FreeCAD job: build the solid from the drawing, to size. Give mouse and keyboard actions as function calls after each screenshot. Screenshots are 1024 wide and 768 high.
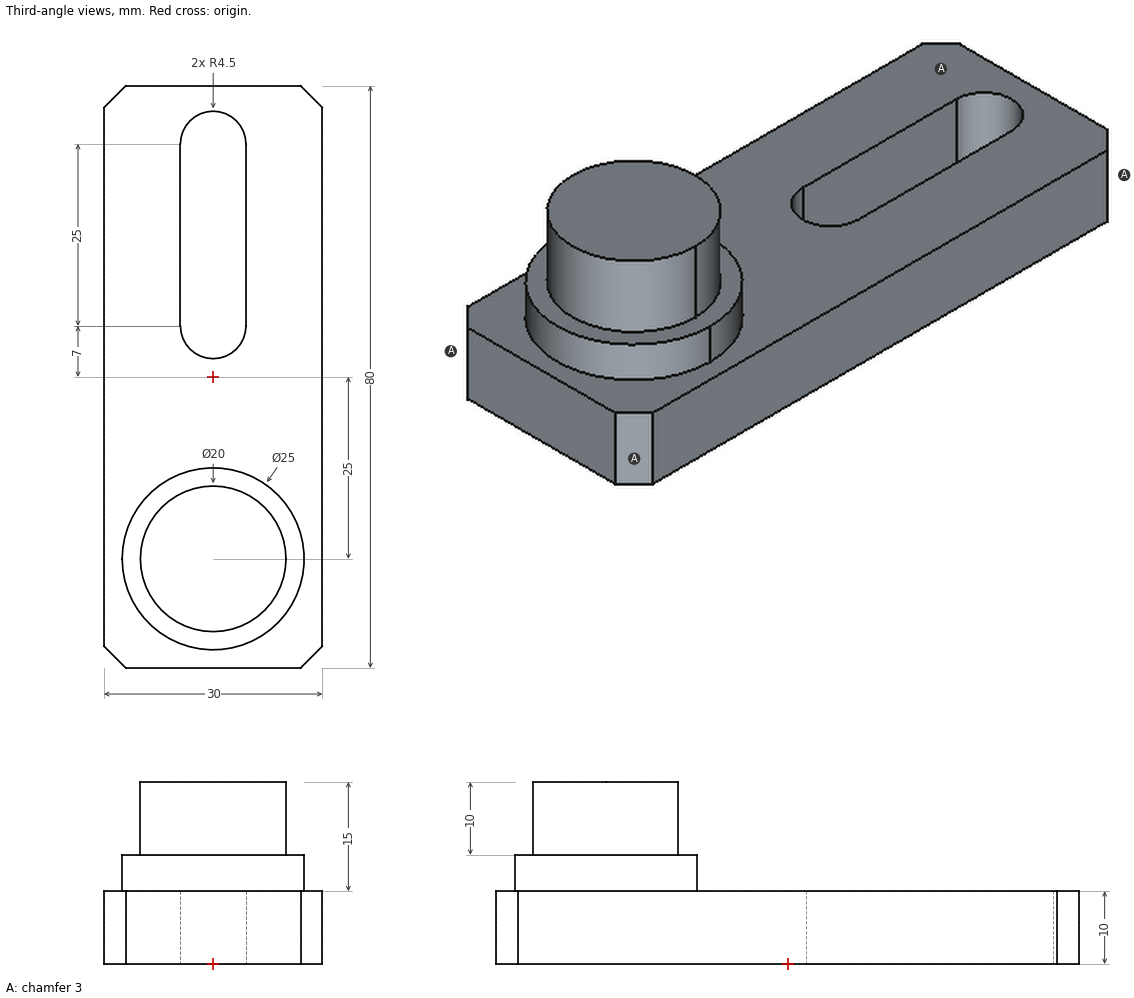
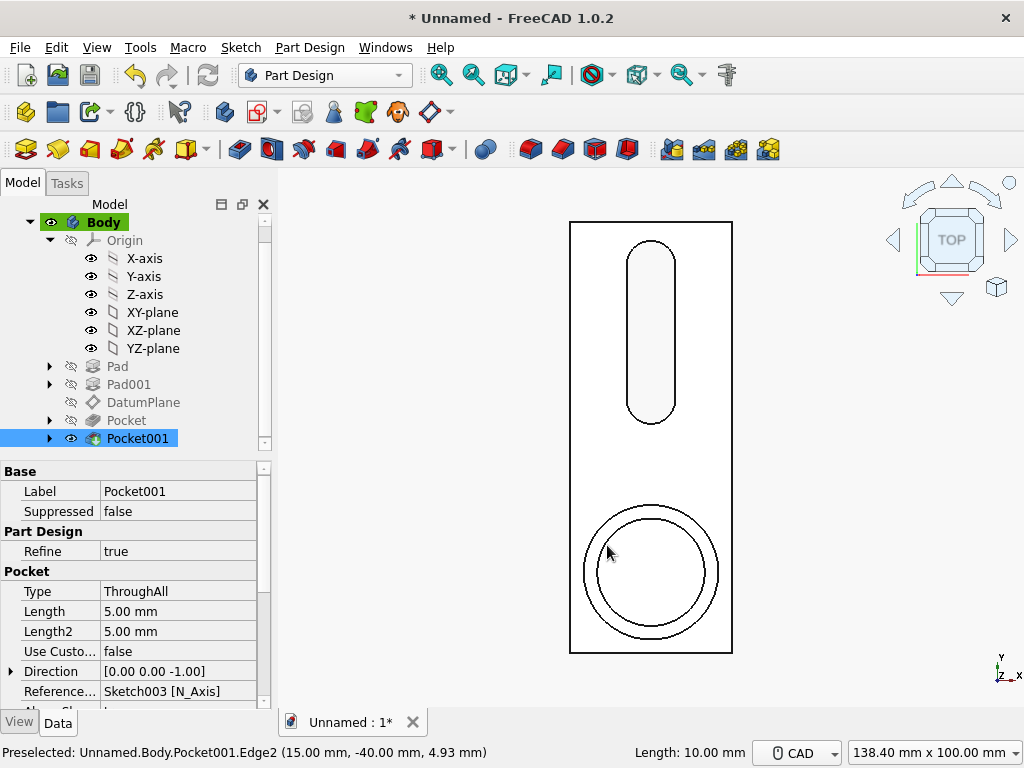
key(1)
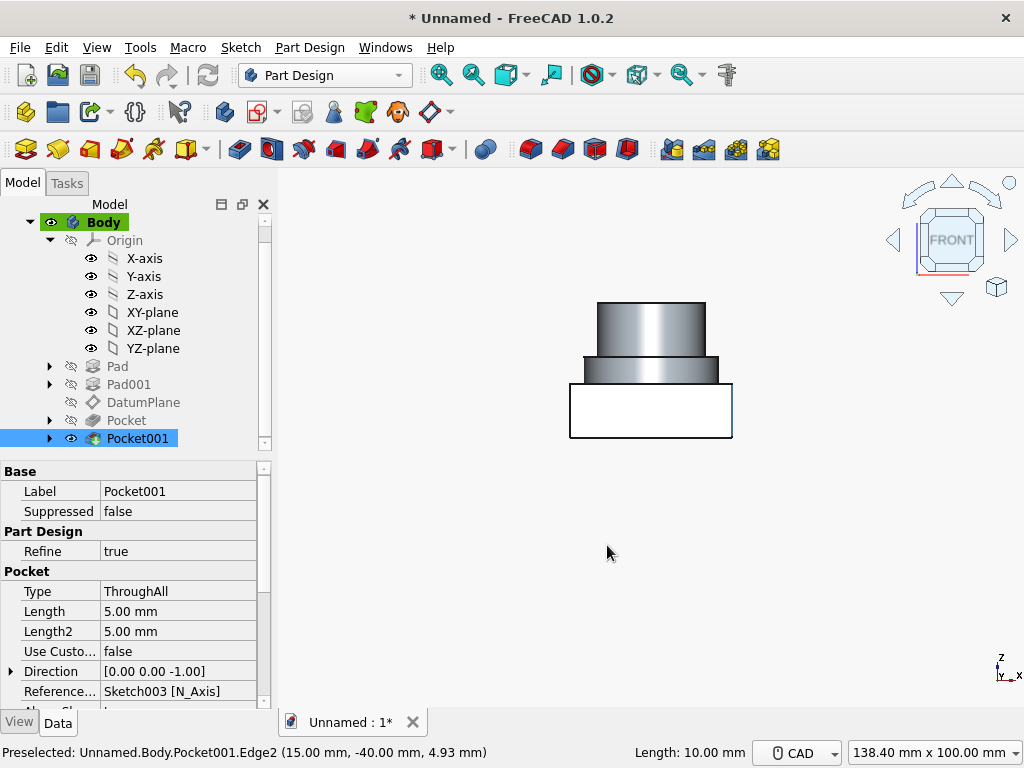
click(442, 76)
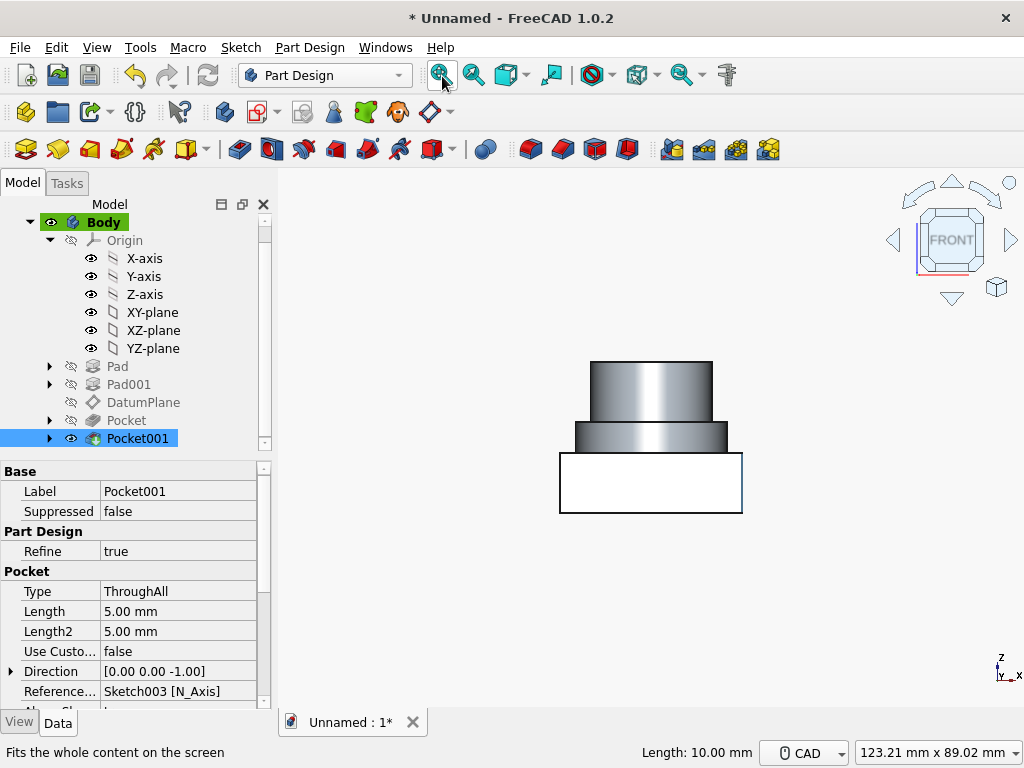
click(560, 482, ctrl)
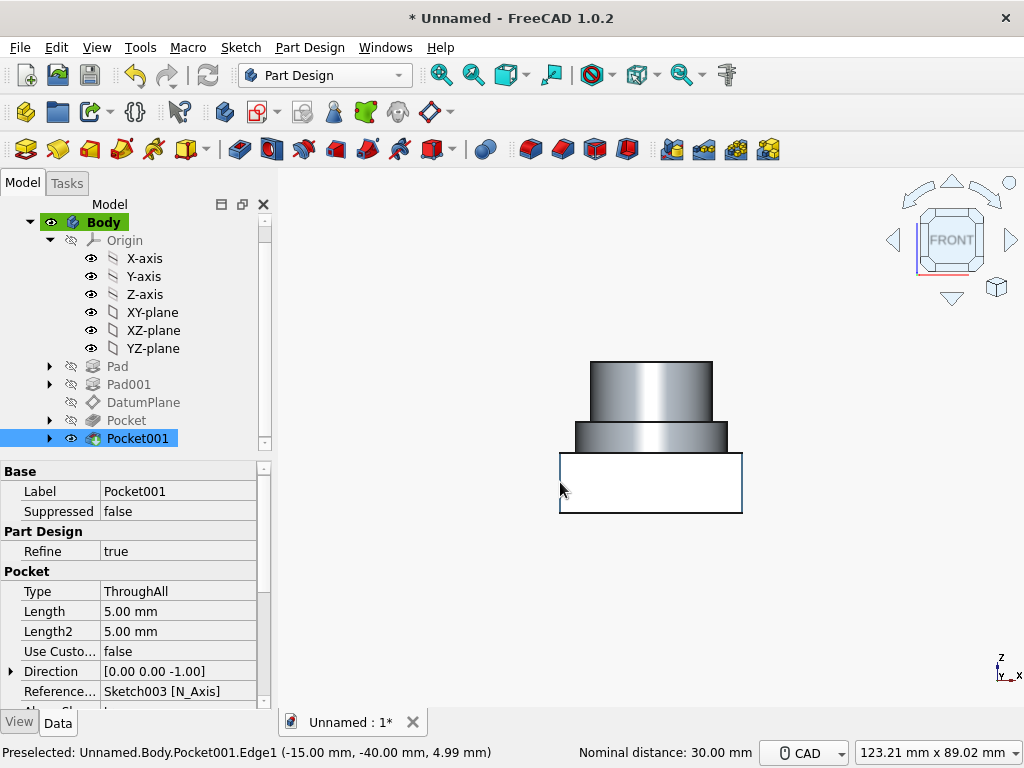
key(3)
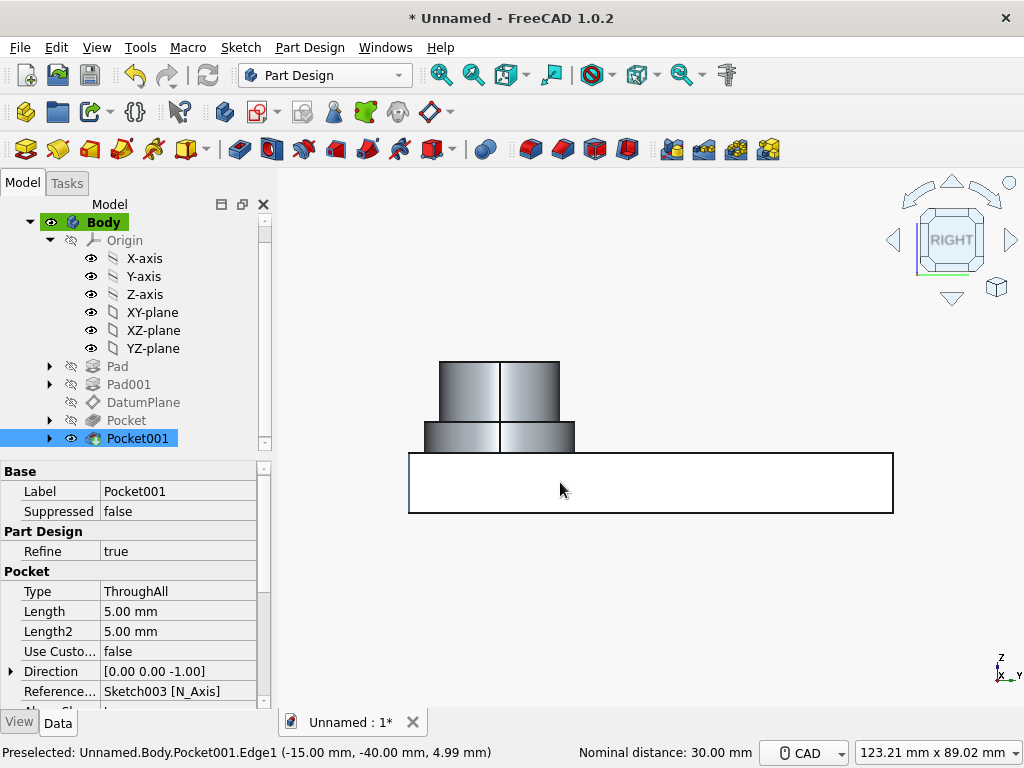
click(893, 482, ctrl)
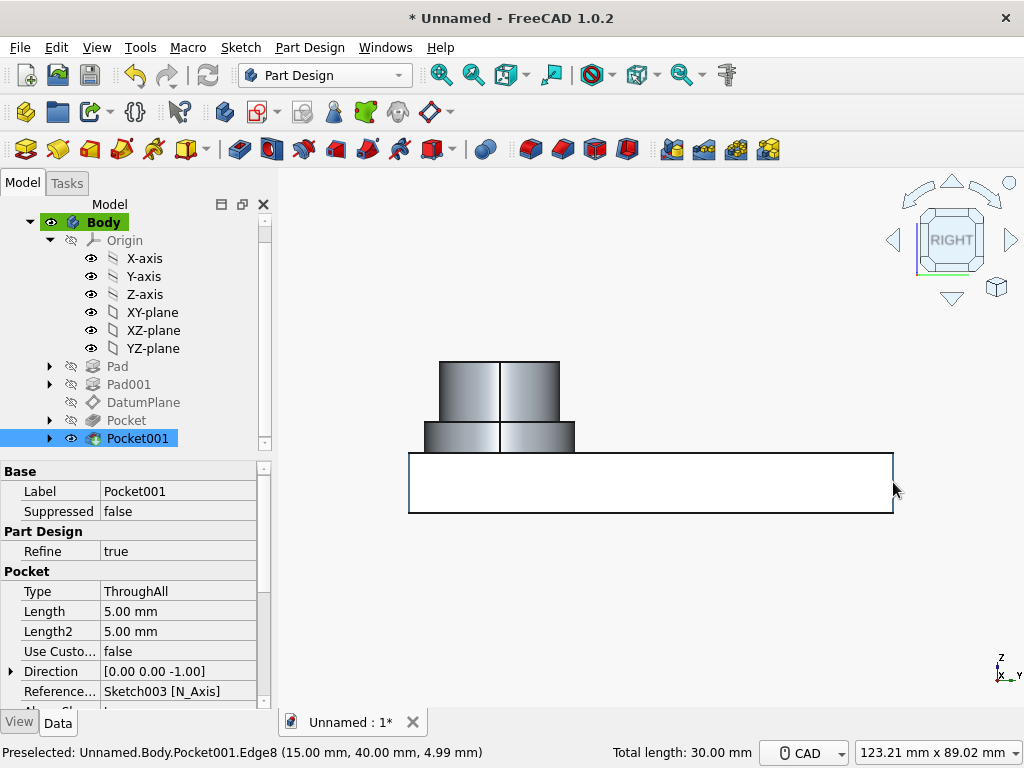
key(5)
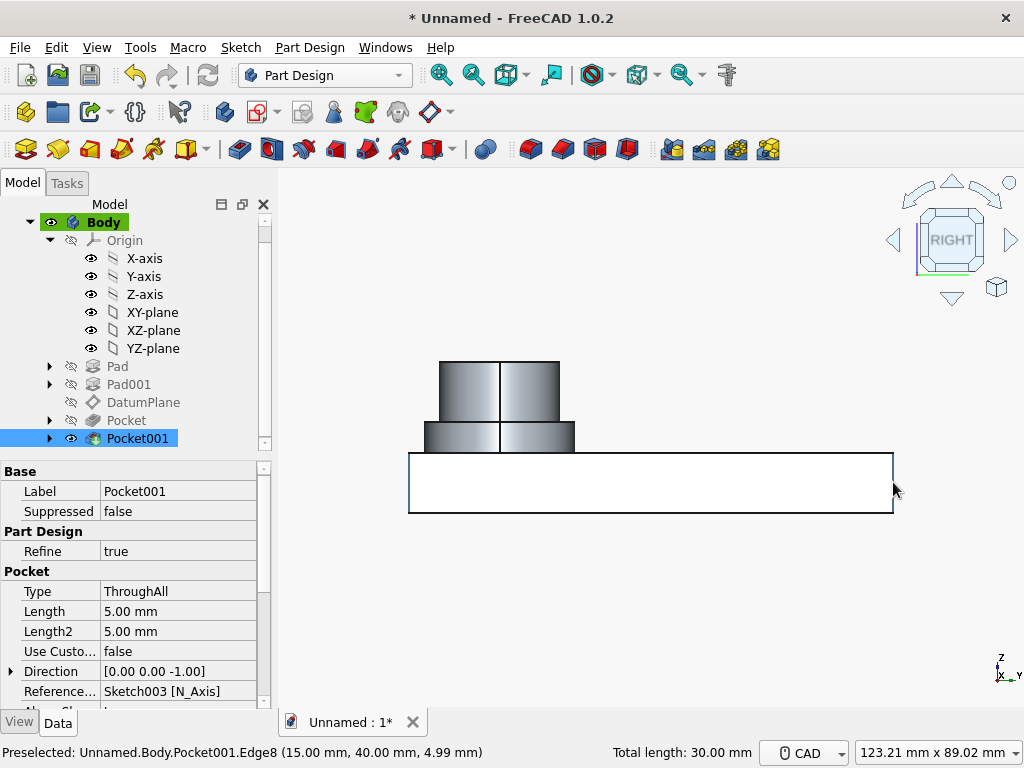
key(4)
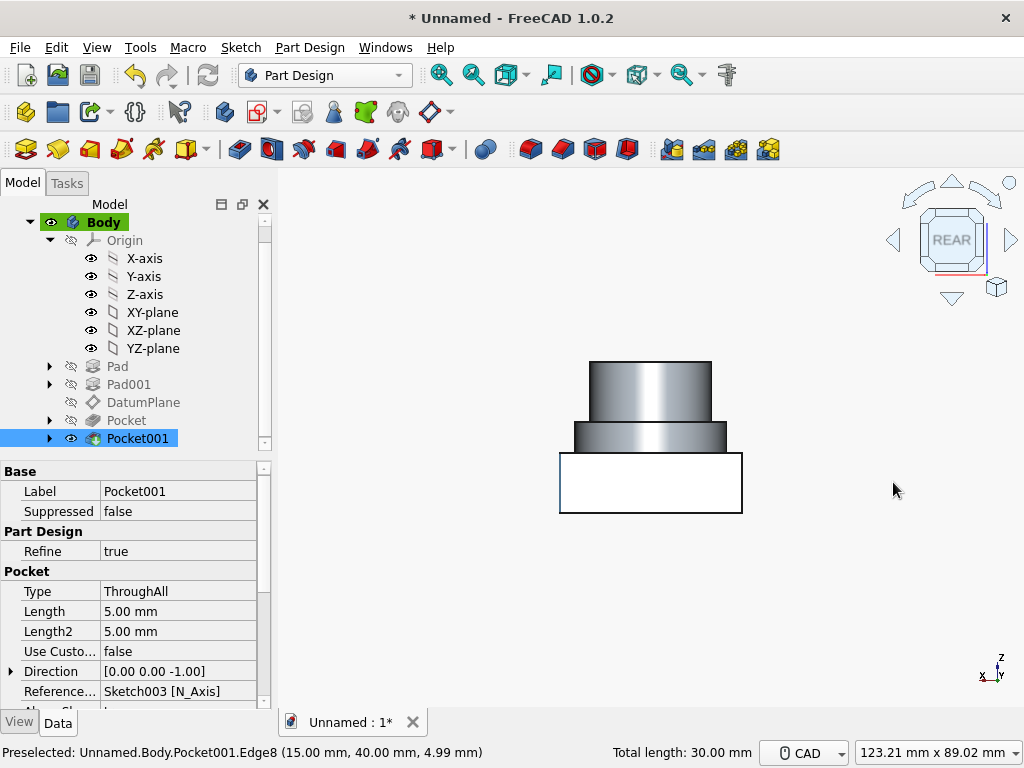
click(442, 76)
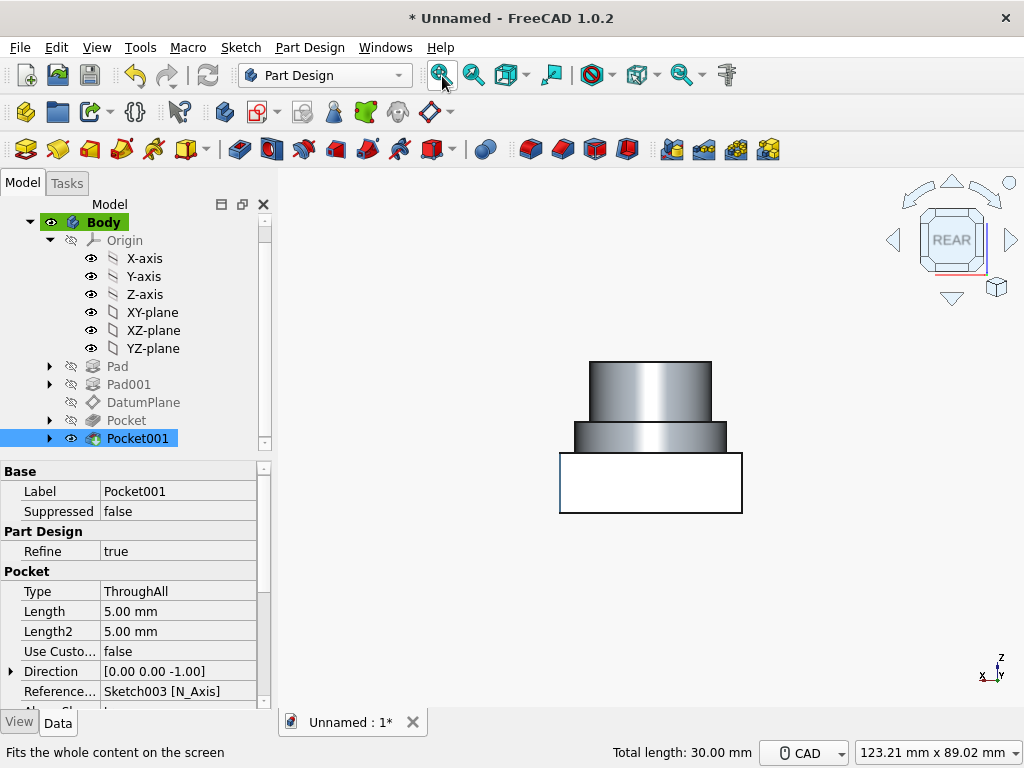
click(742, 482, ctrl)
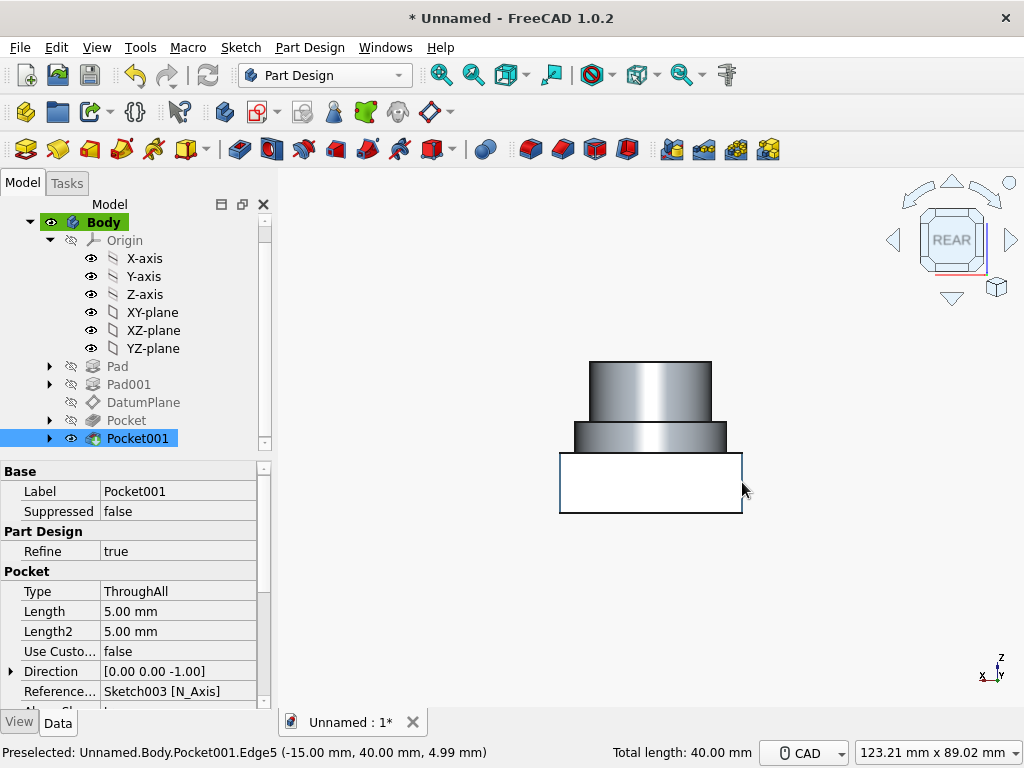
click(564, 150)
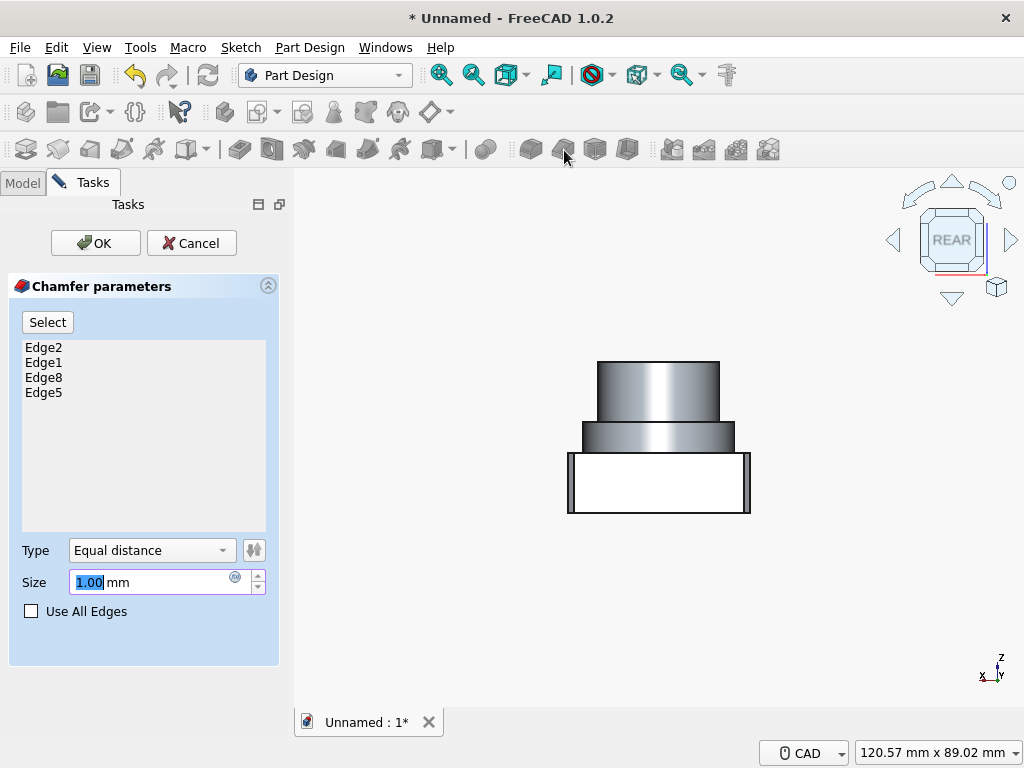
text(3)
key(Tab)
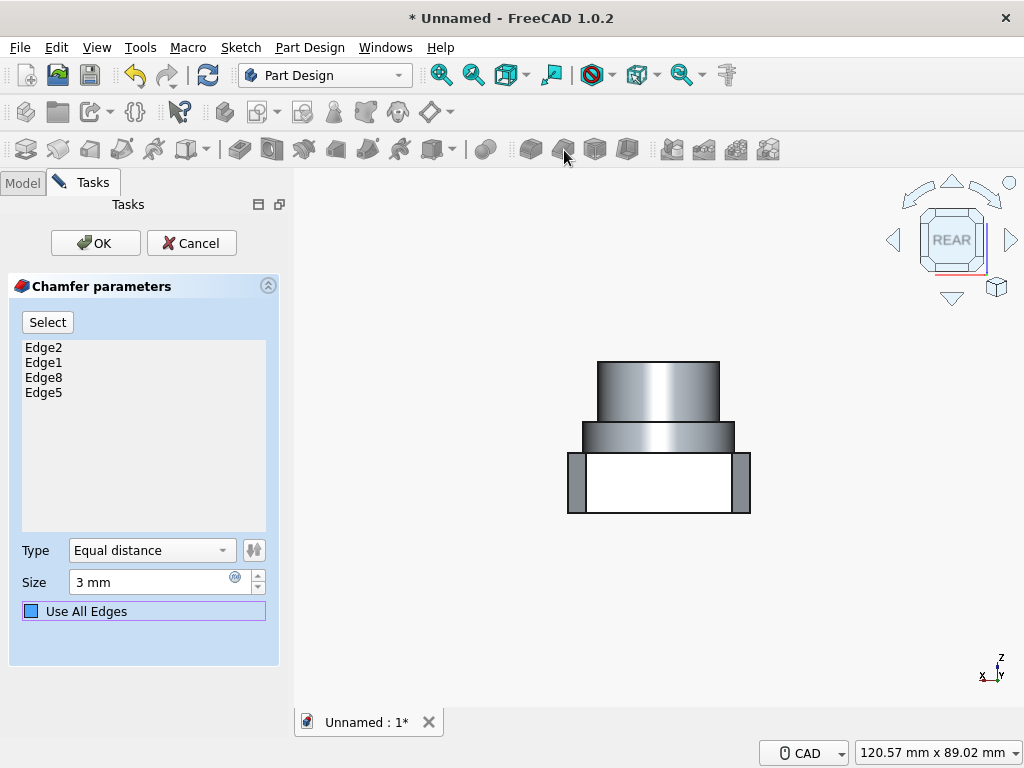
click(96, 243)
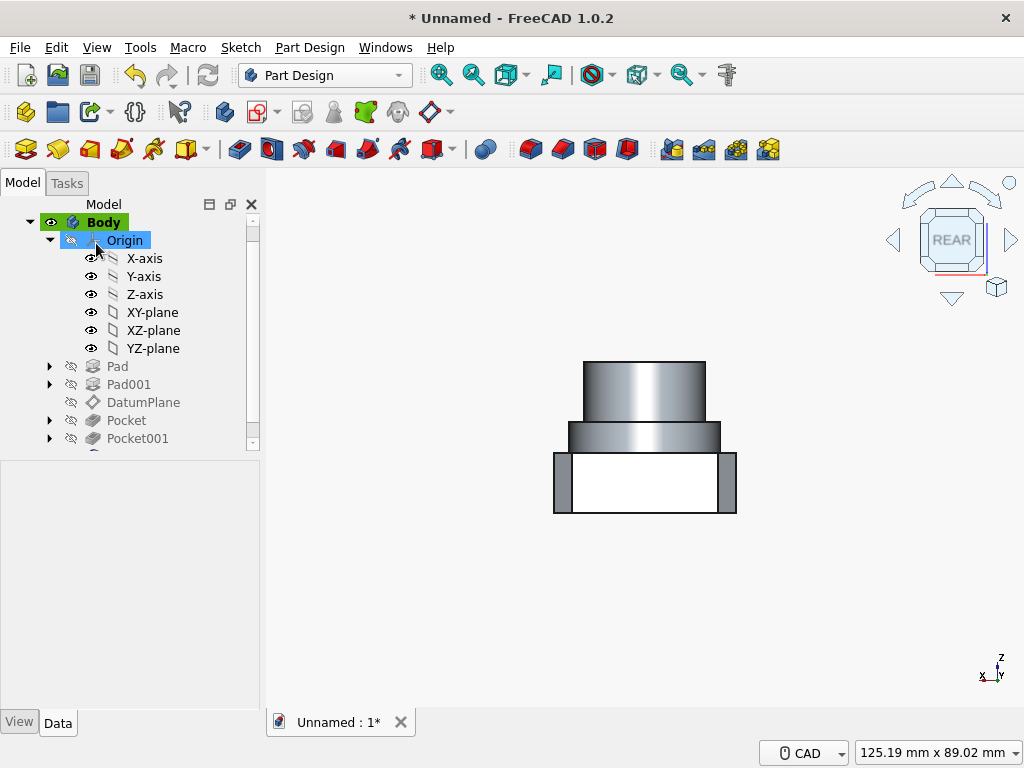
key(0)